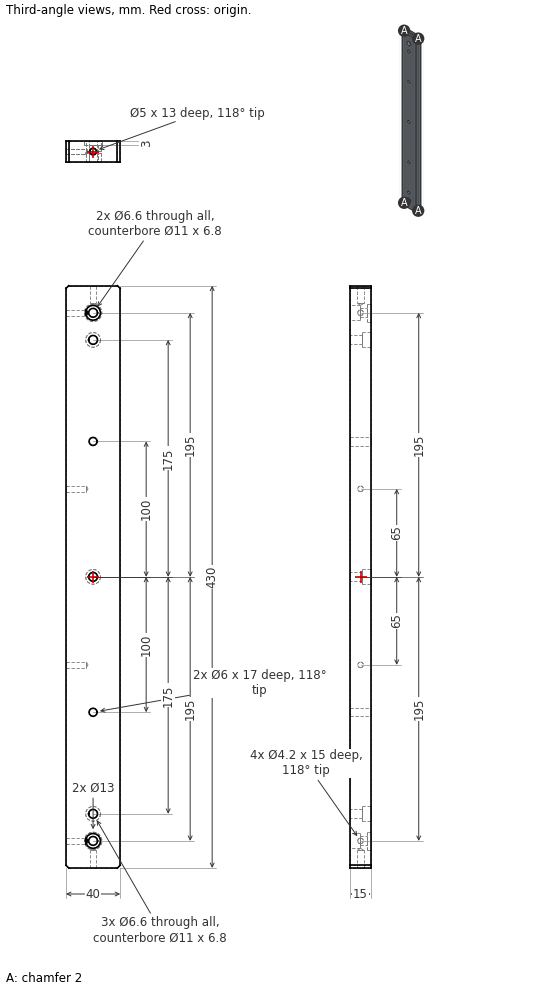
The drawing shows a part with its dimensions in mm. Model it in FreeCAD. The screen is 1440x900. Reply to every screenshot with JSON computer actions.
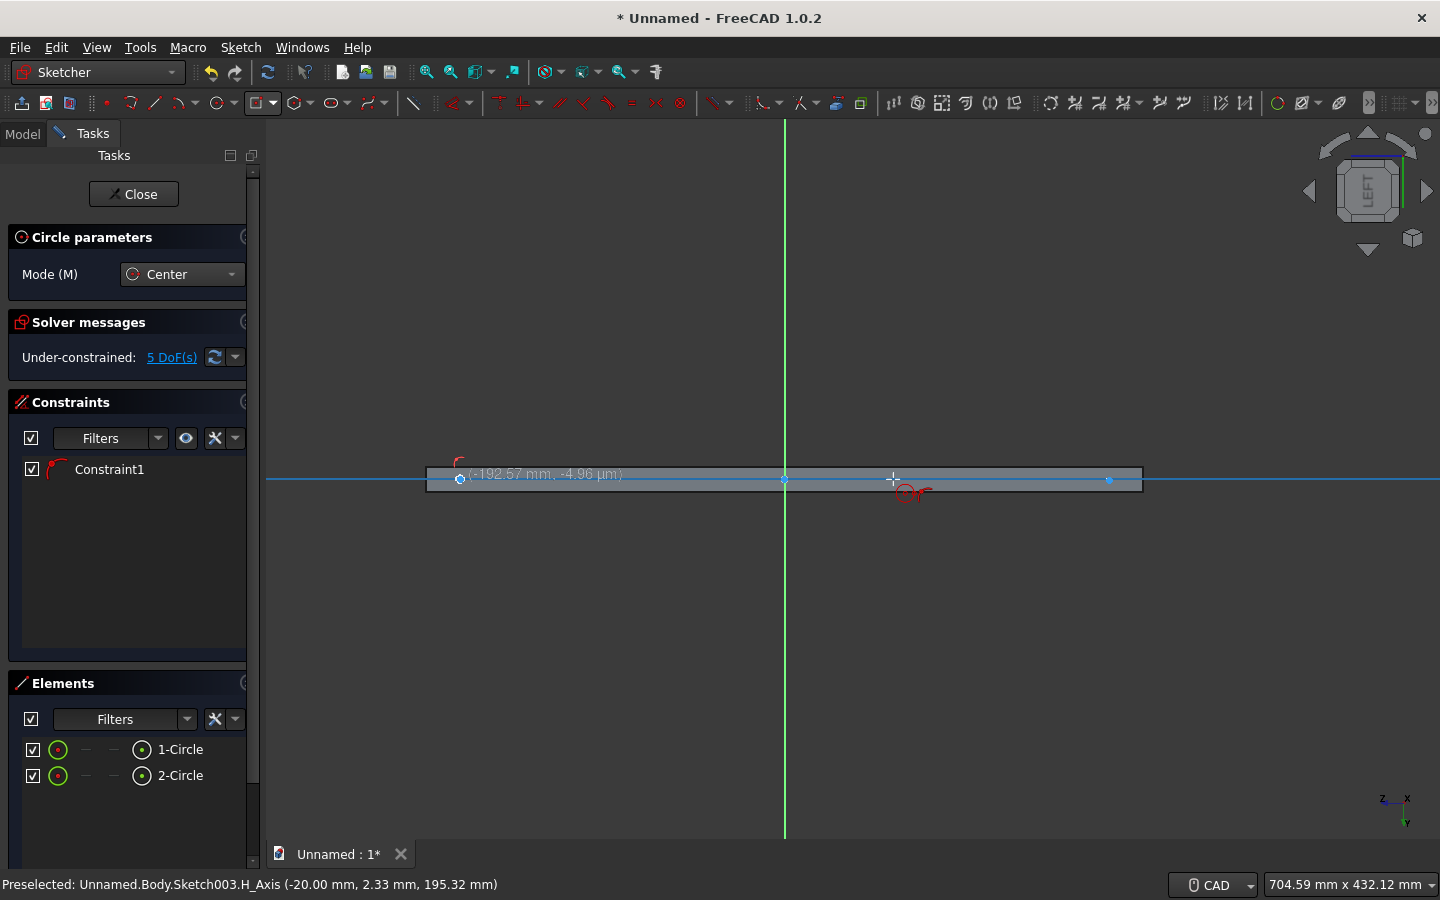
{"action": "left_click", "coordinate": [893, 479]}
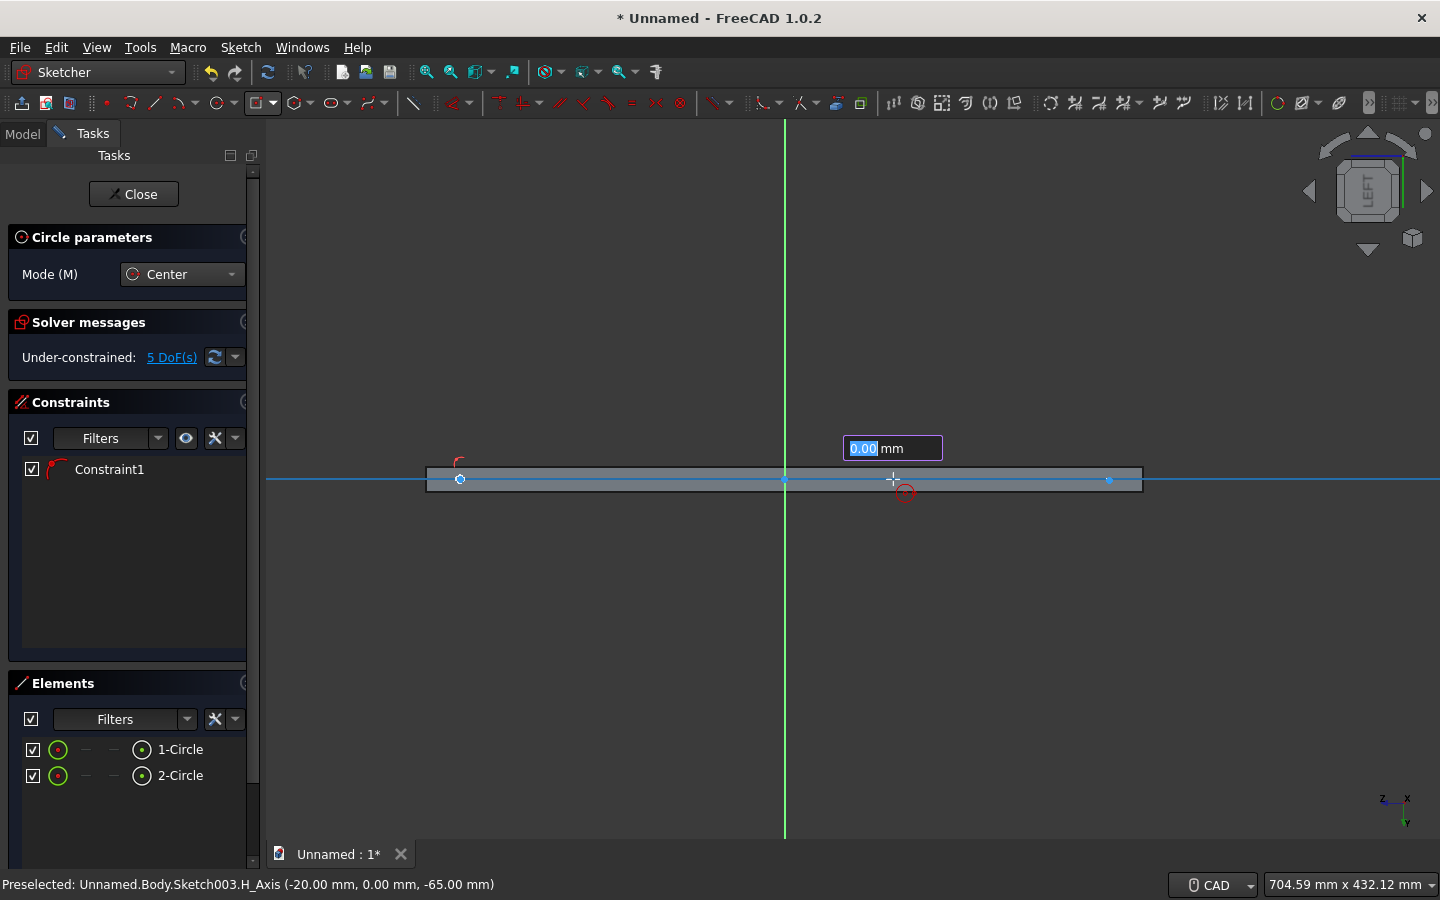
{"action": "scroll", "coordinate": [892, 482], "scroll_direction": "up", "scroll_amount": 8}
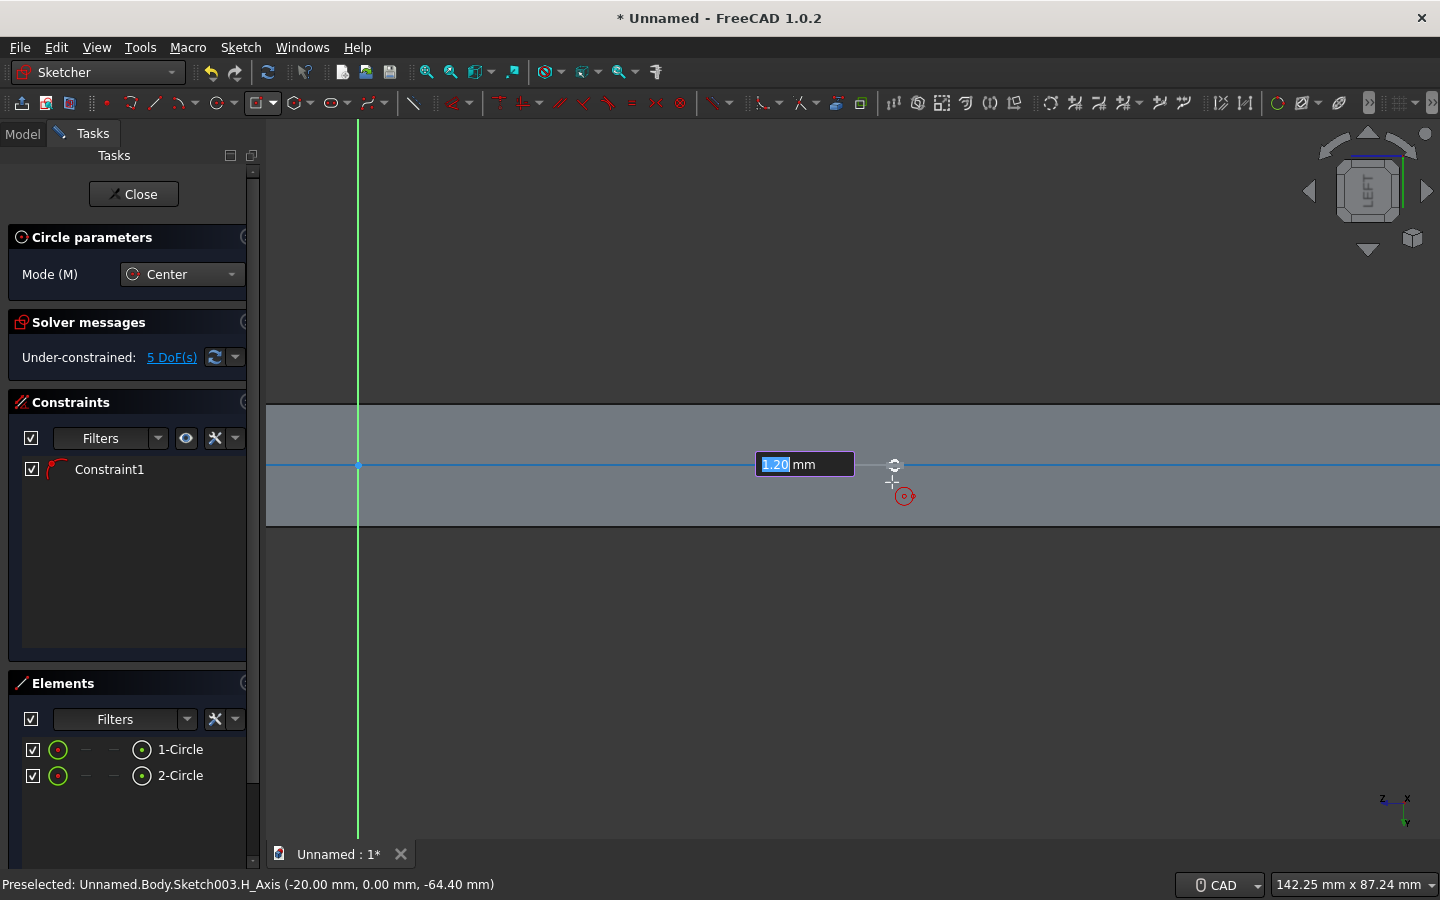
{"action": "left_click", "coordinate": [889, 482]}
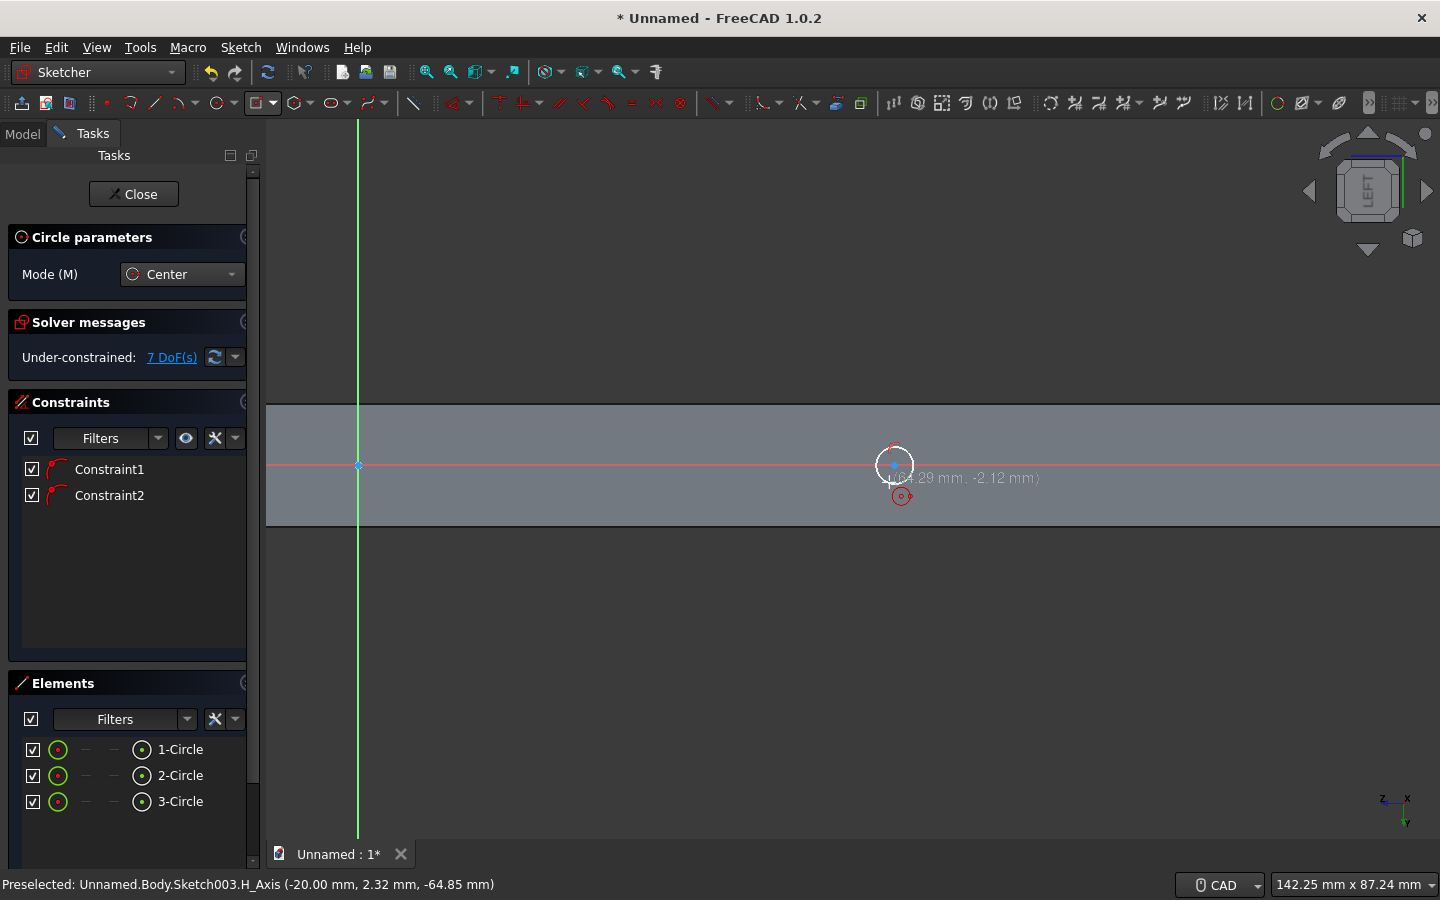
{"action": "scroll", "coordinate": [892, 482], "scroll_direction": "down", "scroll_amount": 8}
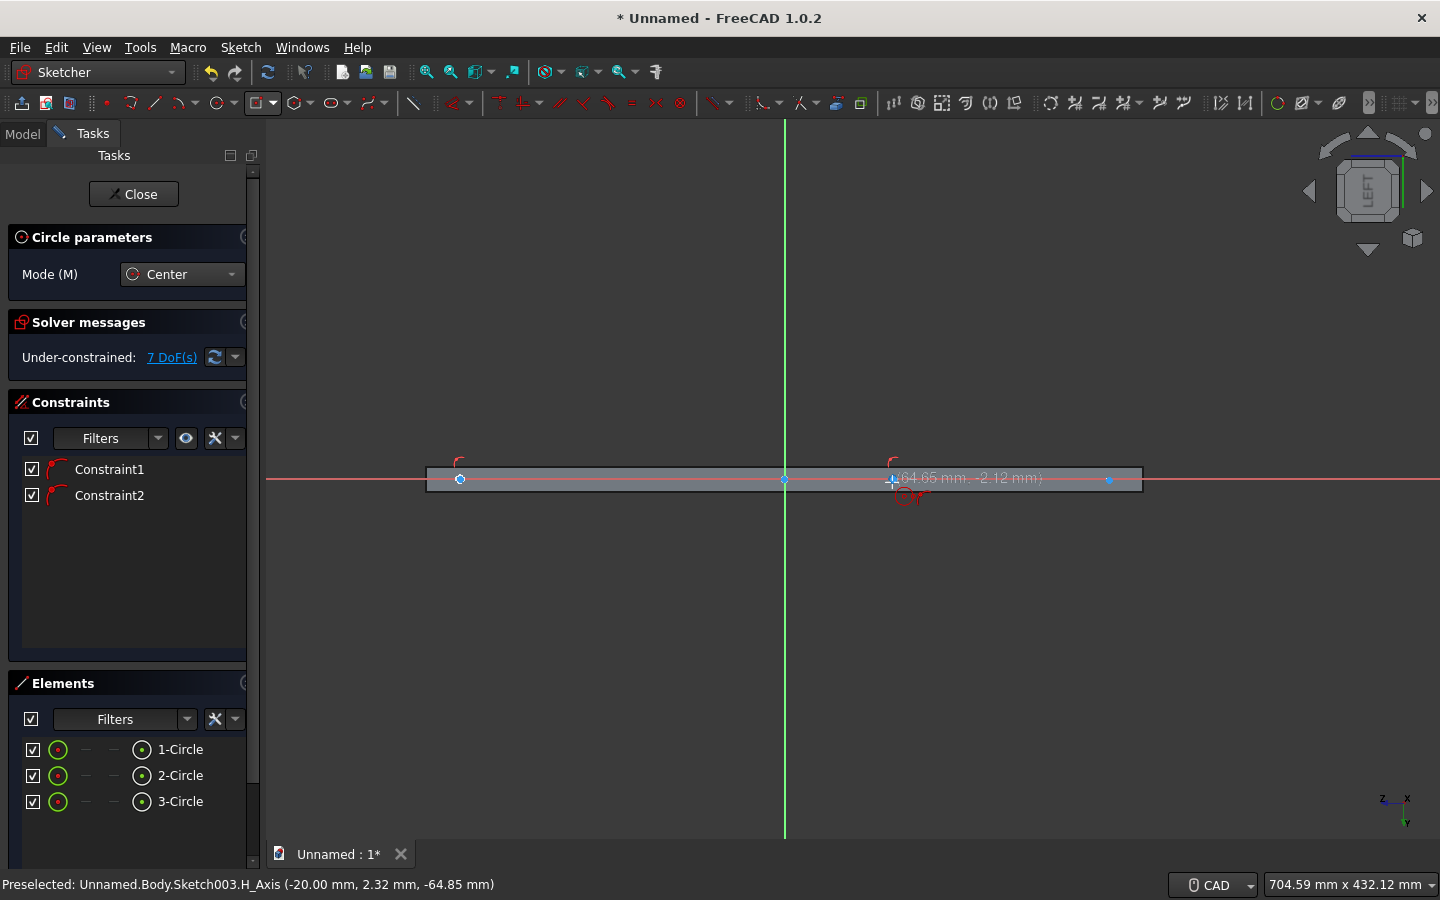
{"action": "scroll", "coordinate": [676, 479], "scroll_direction": "up", "scroll_amount": 10}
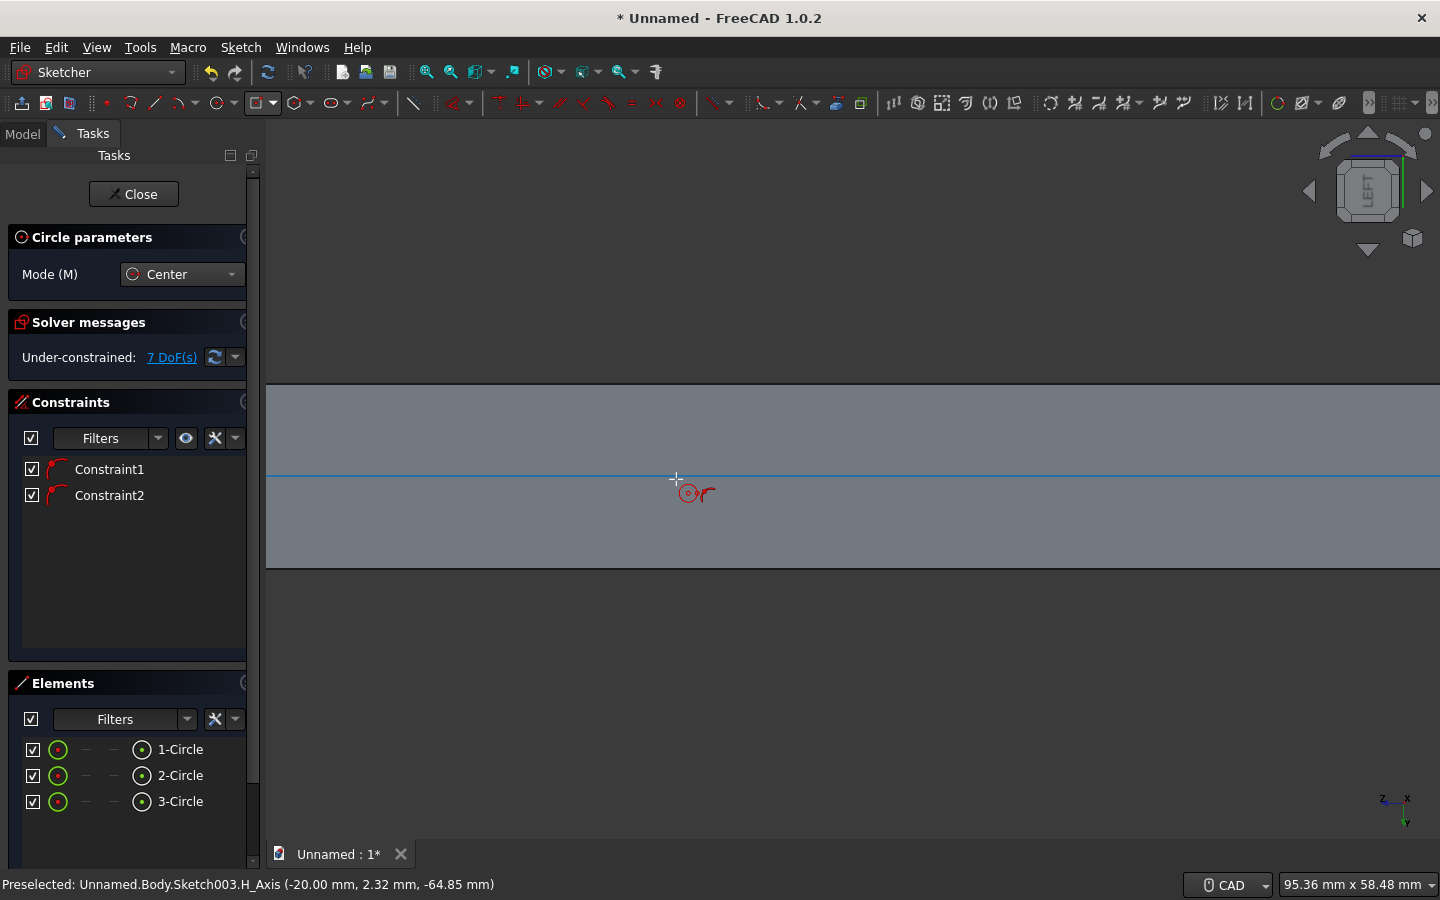
{"action": "scroll", "coordinate": [676, 479], "scroll_direction": "down", "scroll_amount": 10}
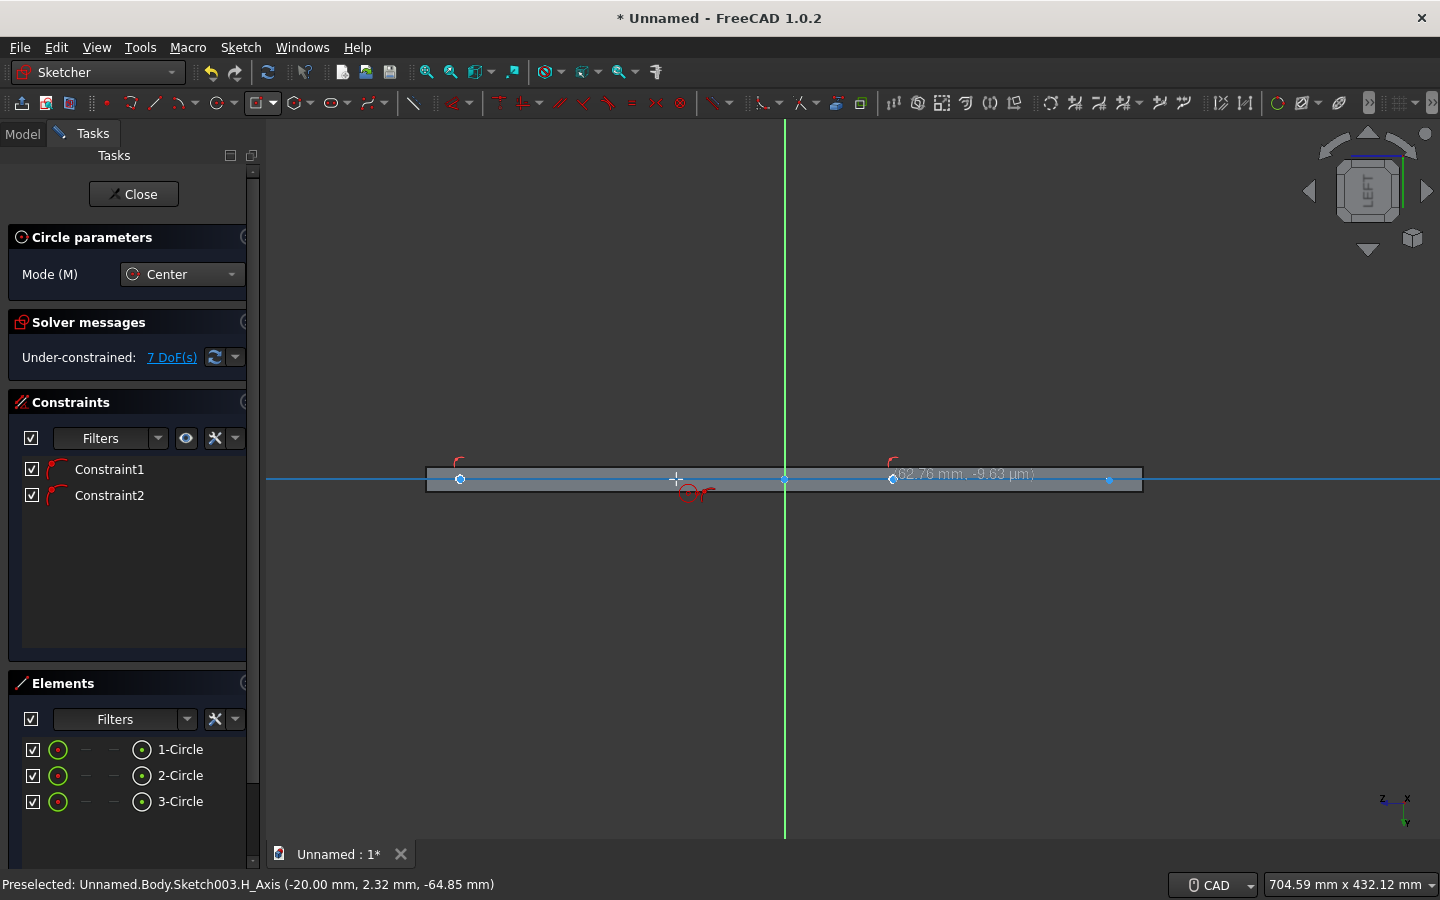
{"action": "left_click", "coordinate": [676, 479]}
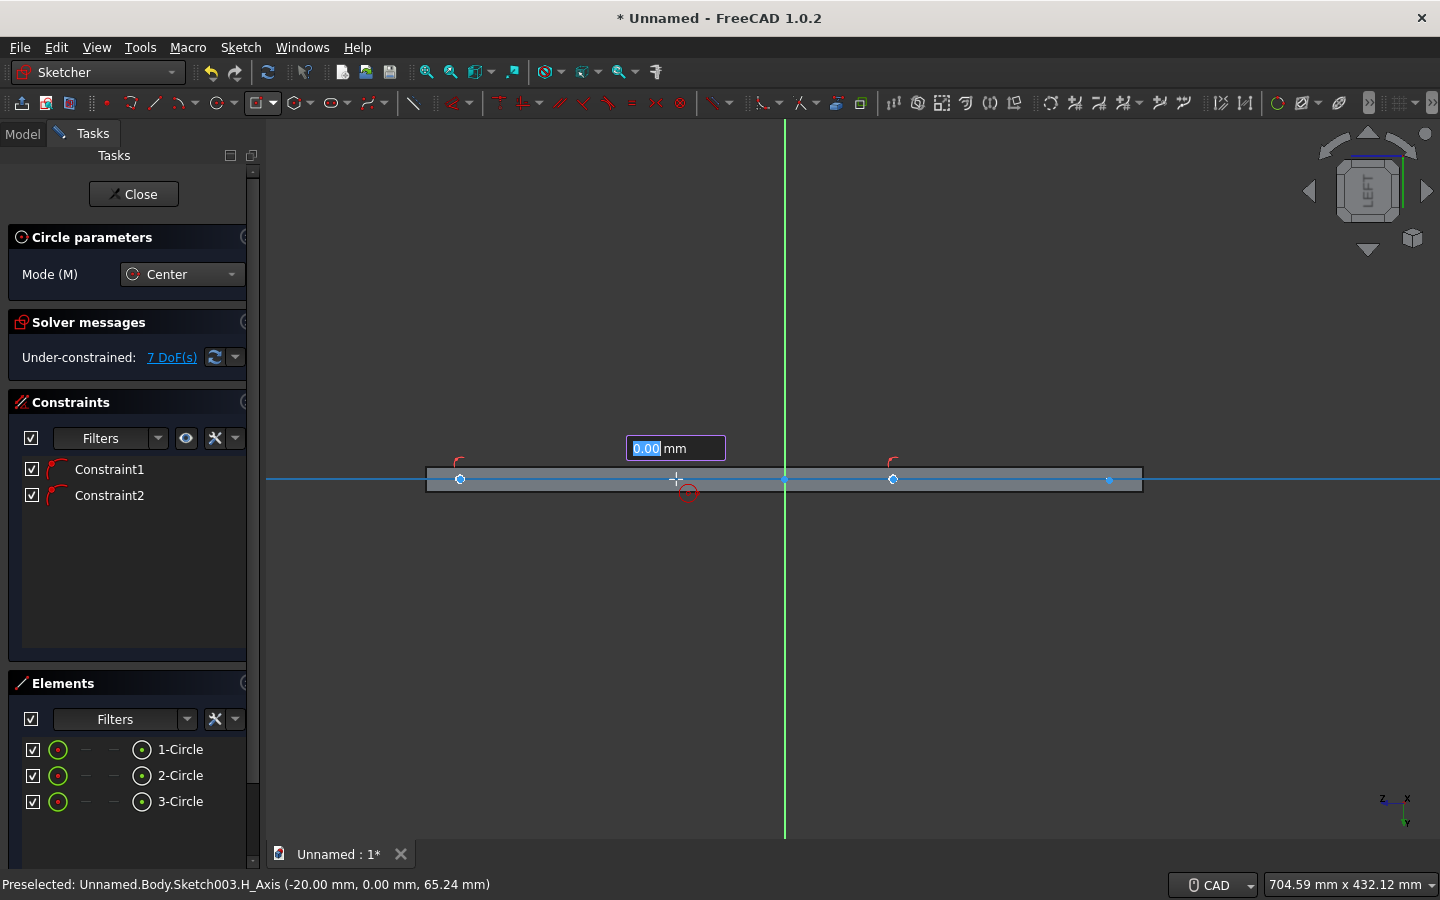
{"action": "scroll", "coordinate": [675, 482], "scroll_direction": "up", "scroll_amount": 8}